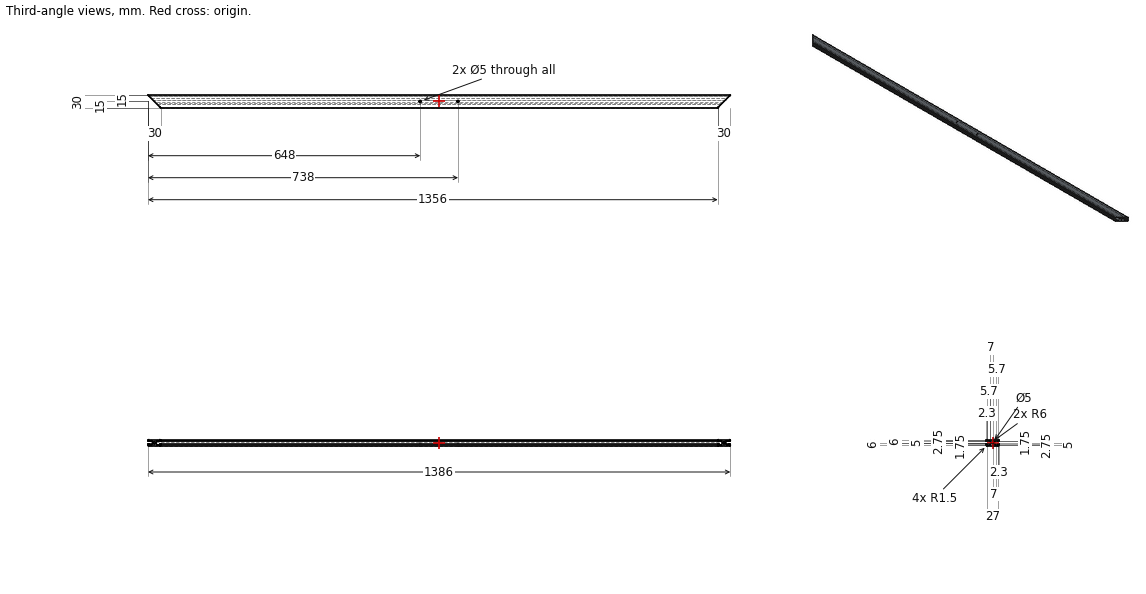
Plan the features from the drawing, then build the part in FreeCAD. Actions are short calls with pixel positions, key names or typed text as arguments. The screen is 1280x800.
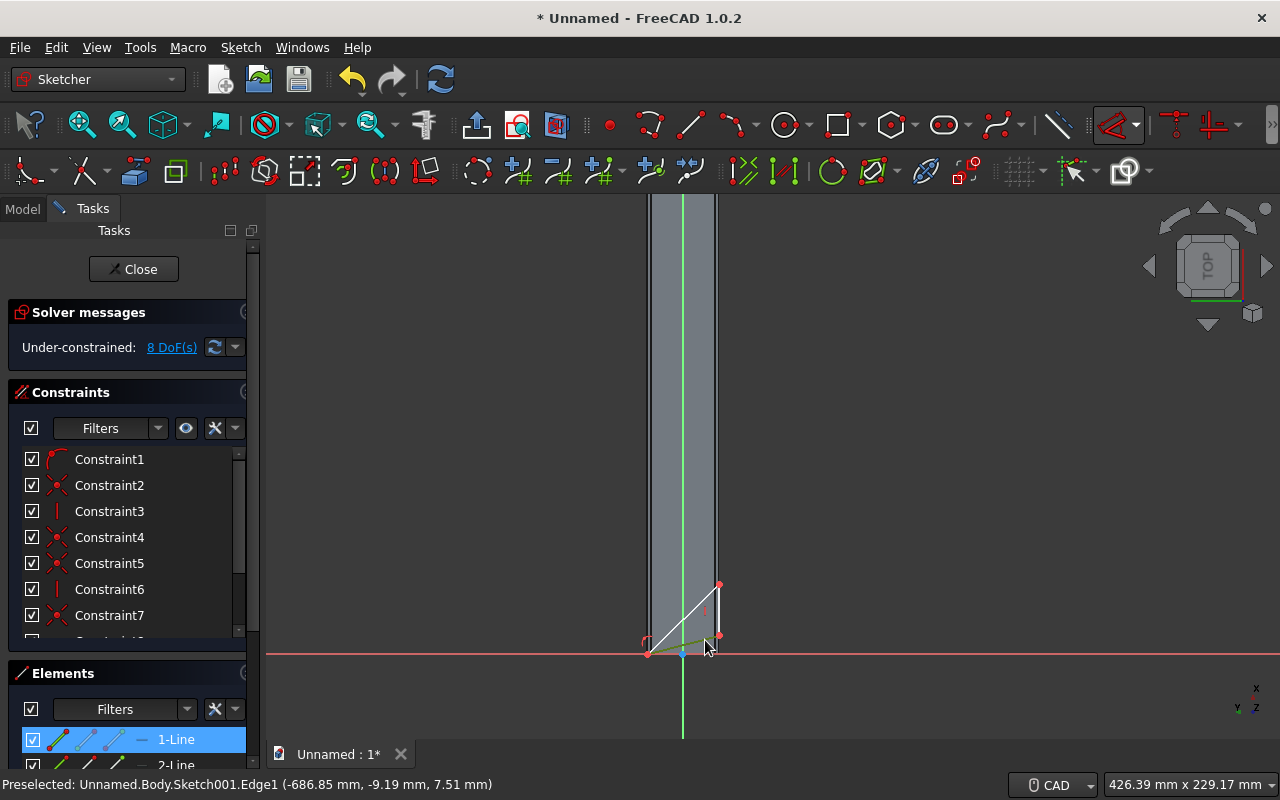
click(1240, 126)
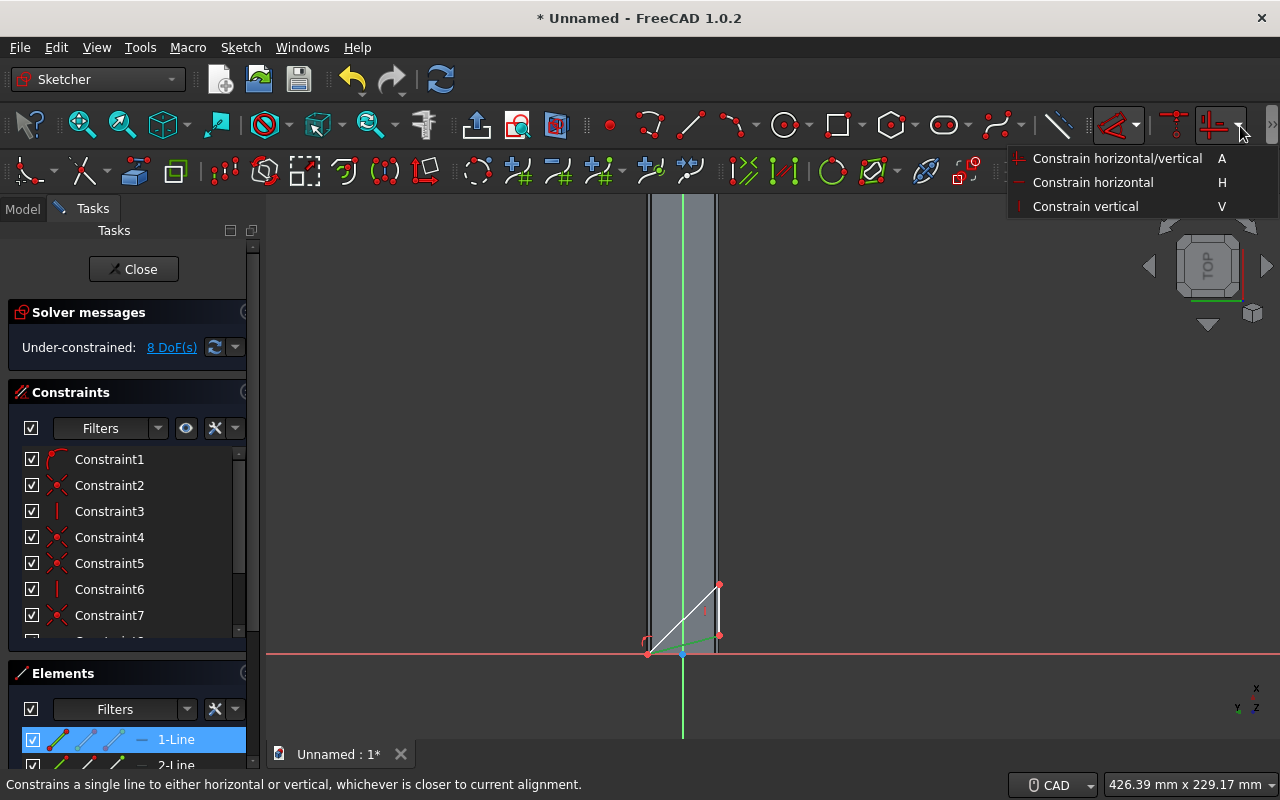
click(1143, 182)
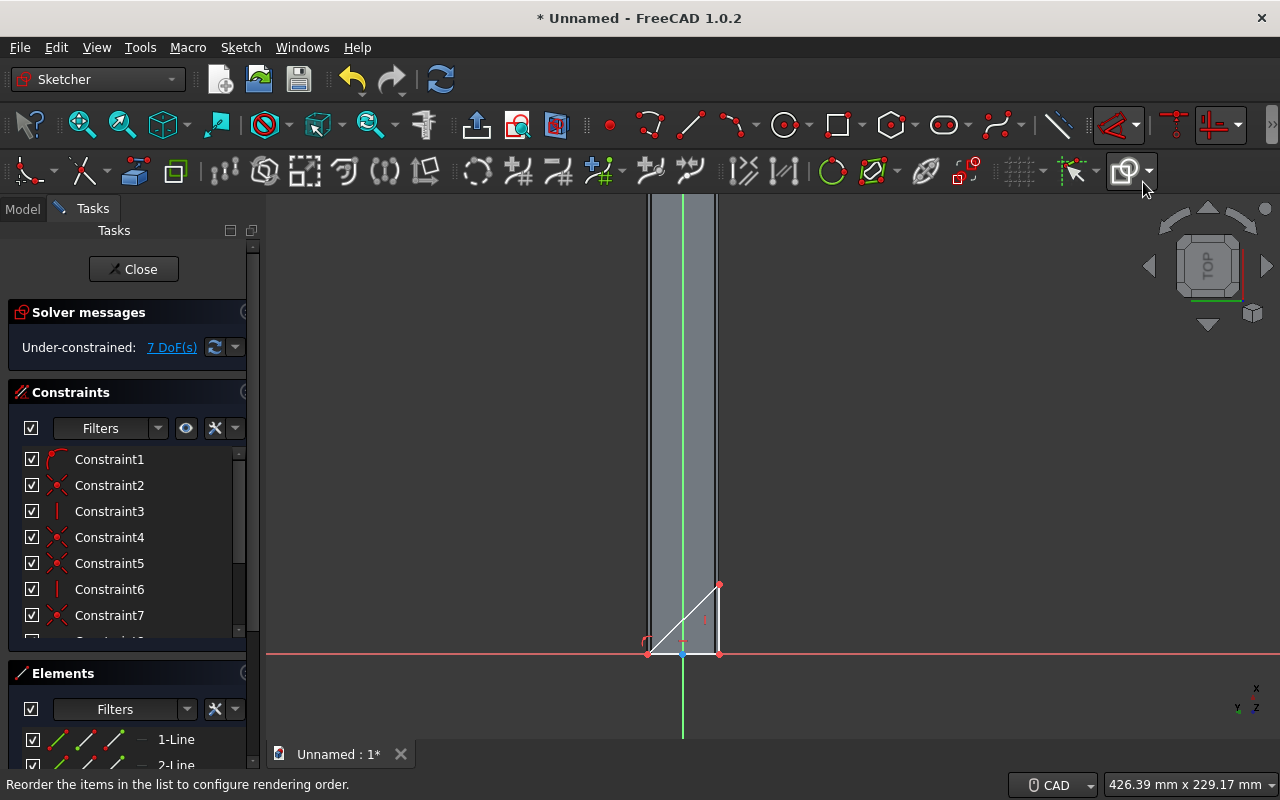
click(669, 654)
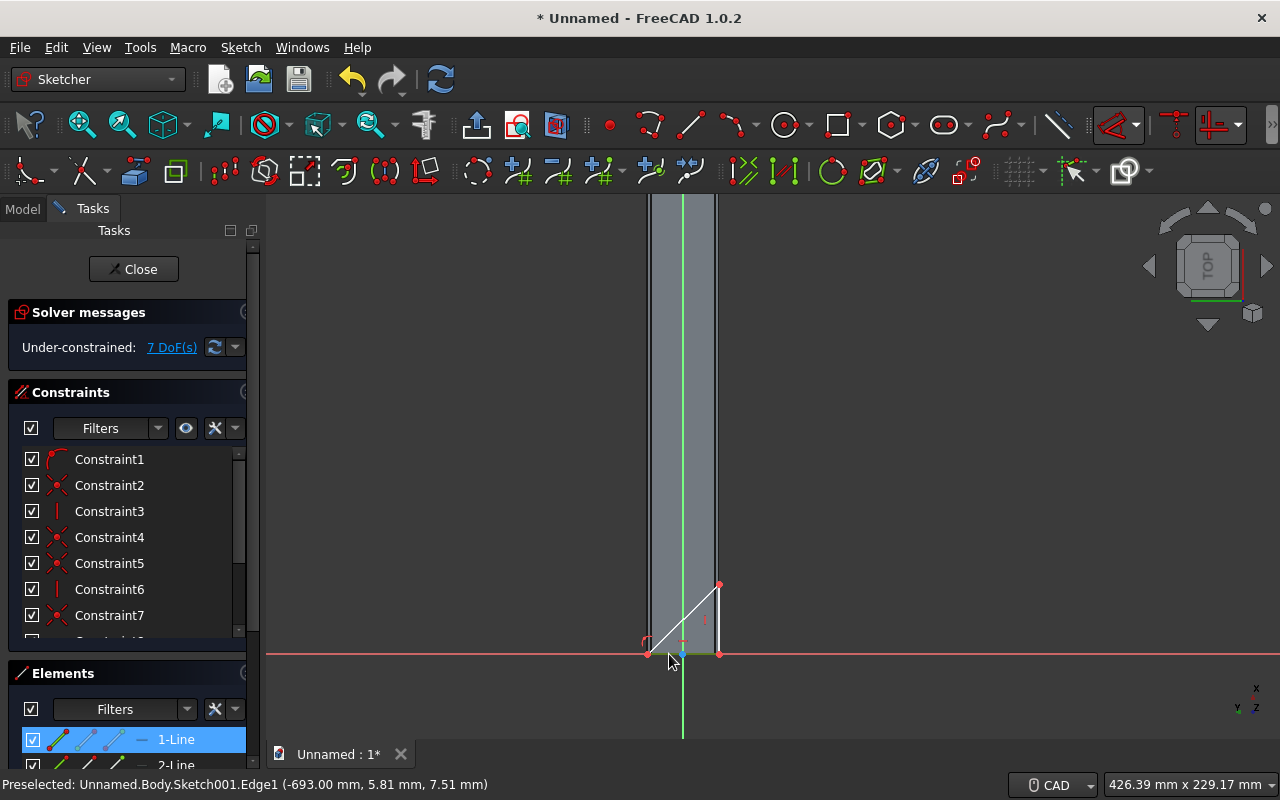
click(1138, 126)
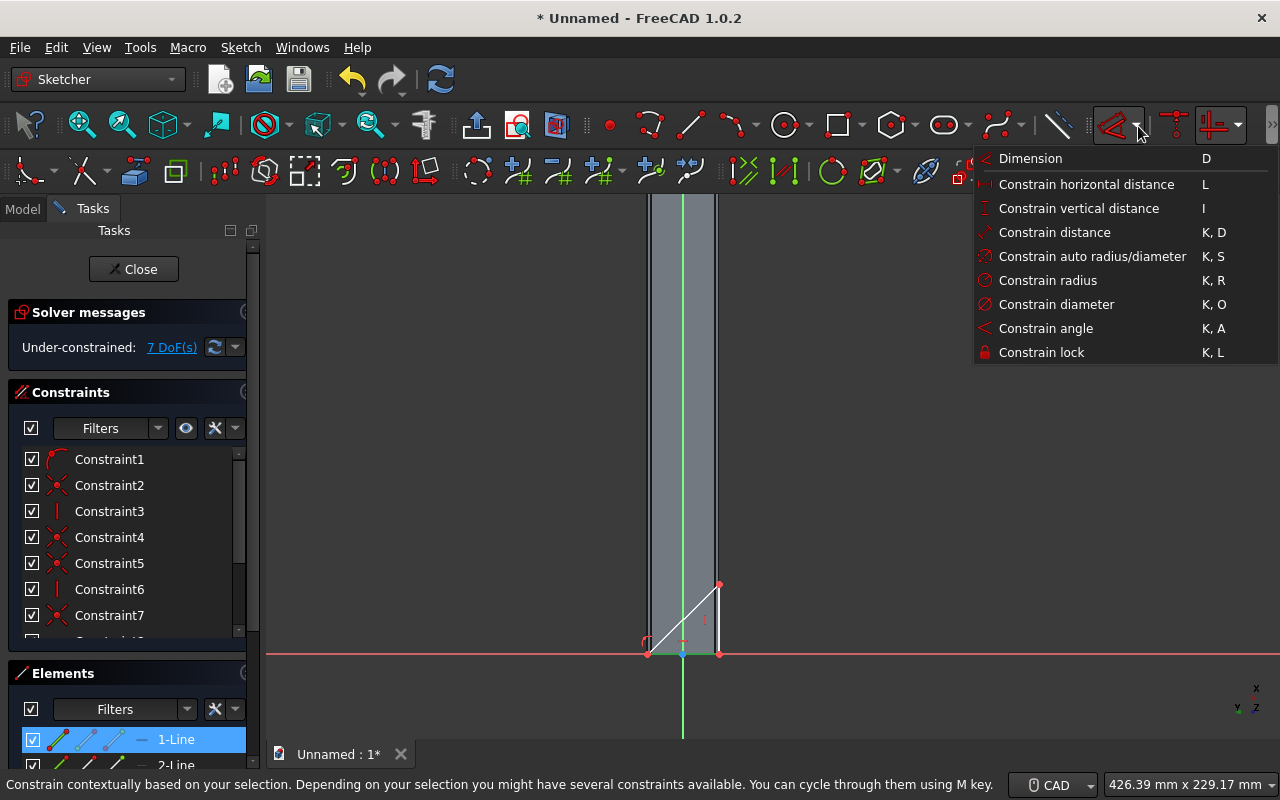
click(1126, 184)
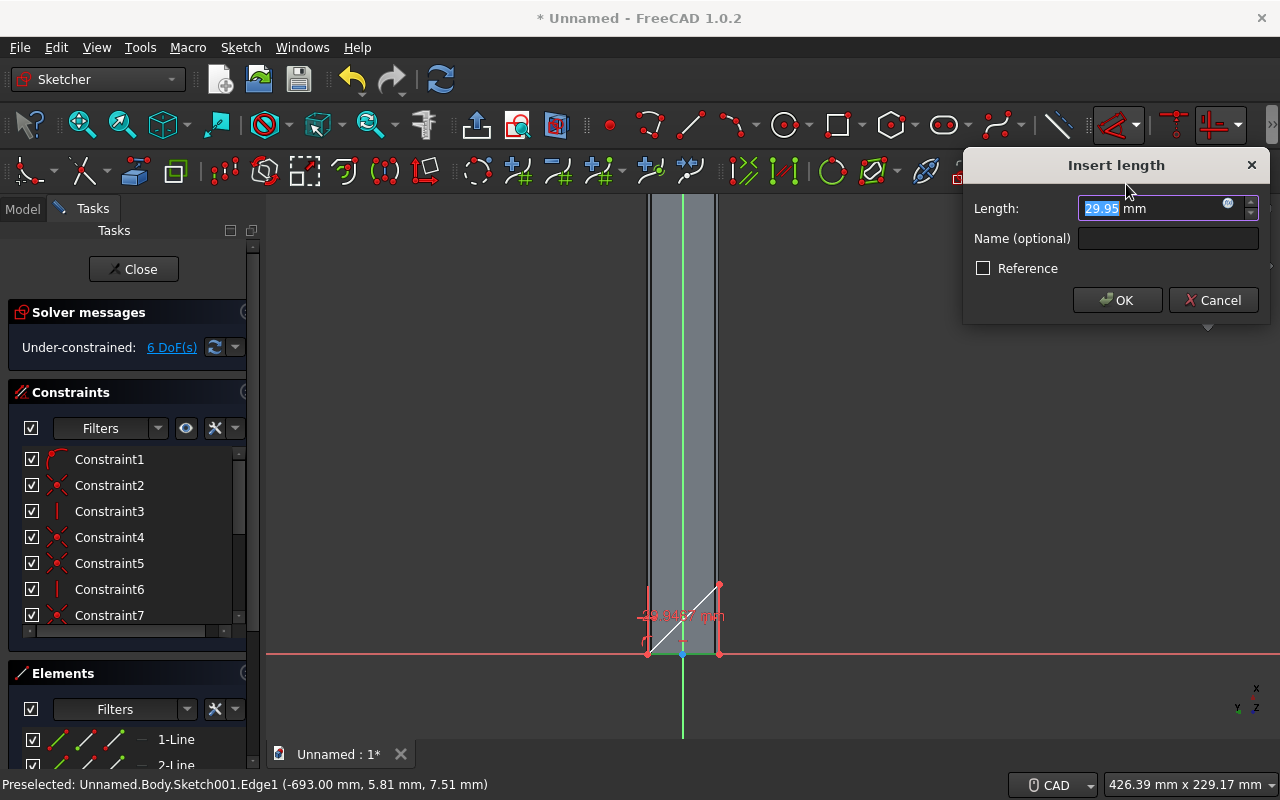
text(30)
key(Return)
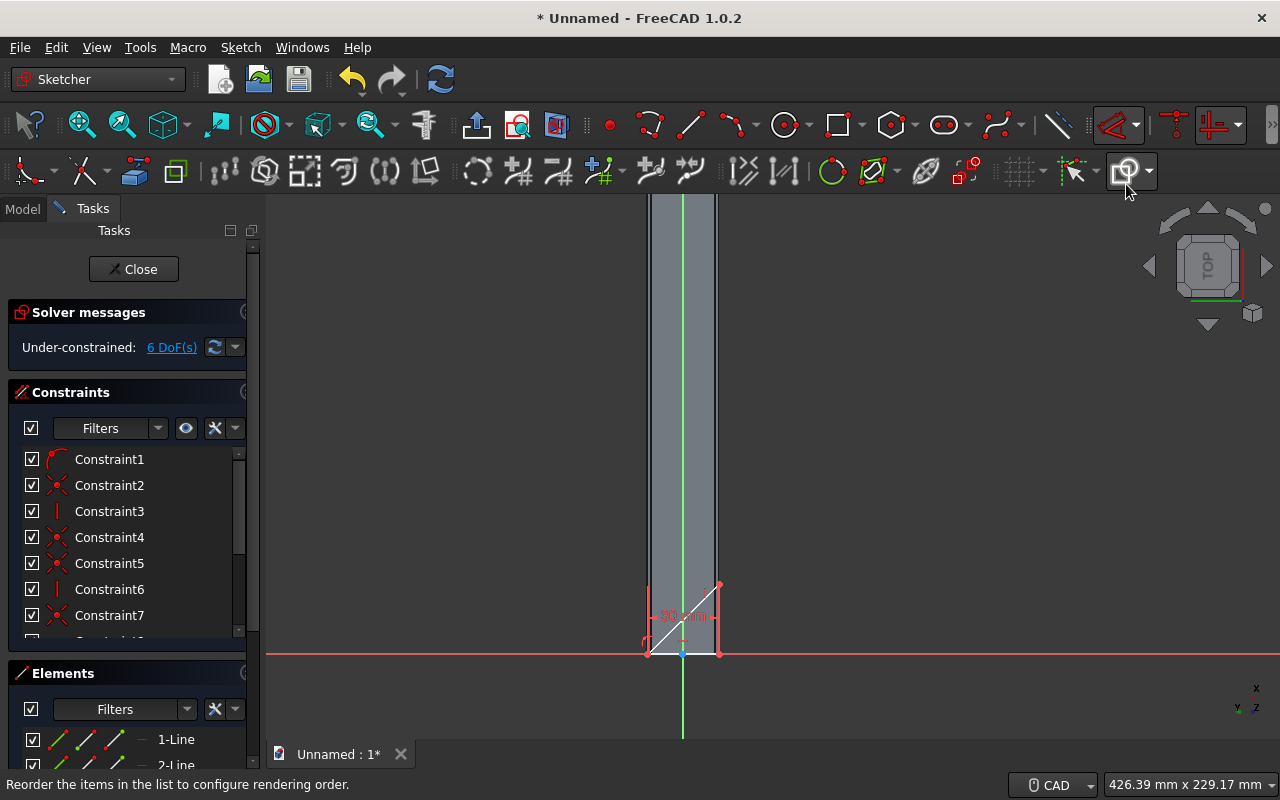
click(719, 633)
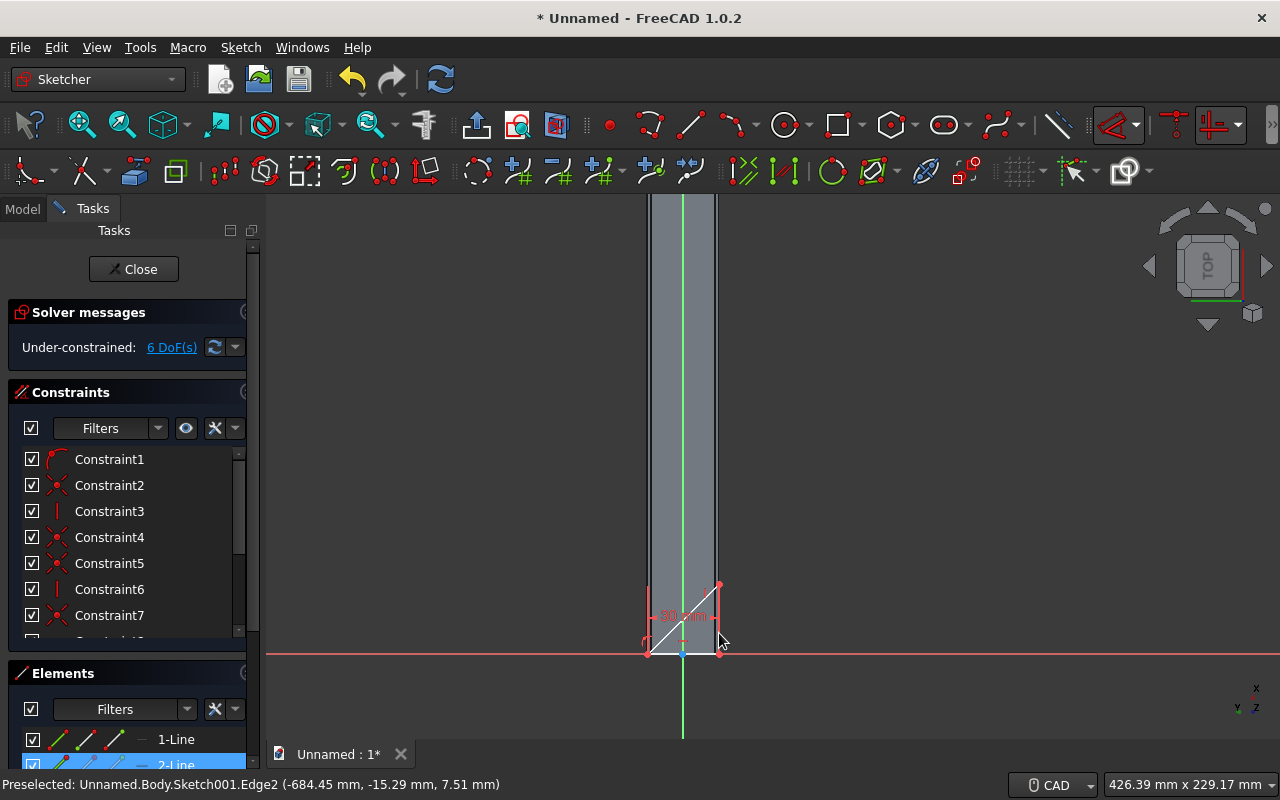
key(i)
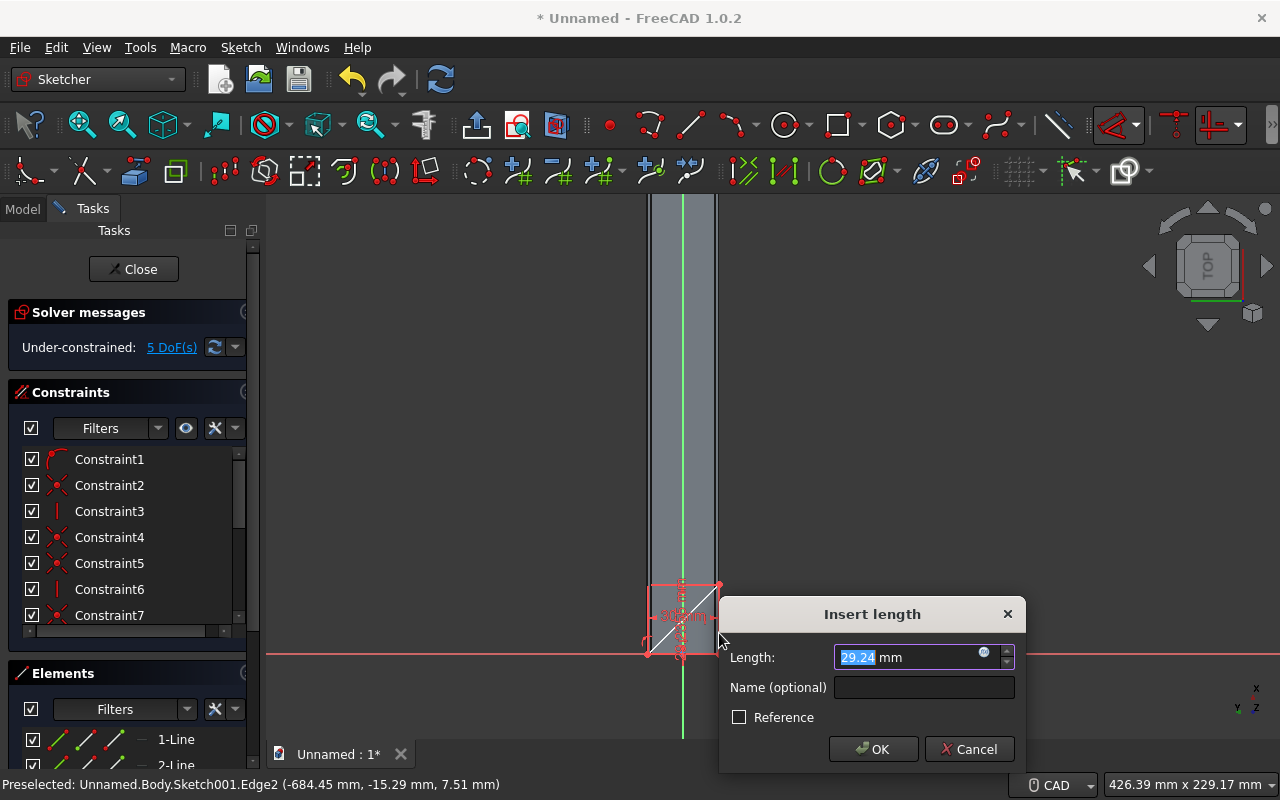
text(30)
key(Return)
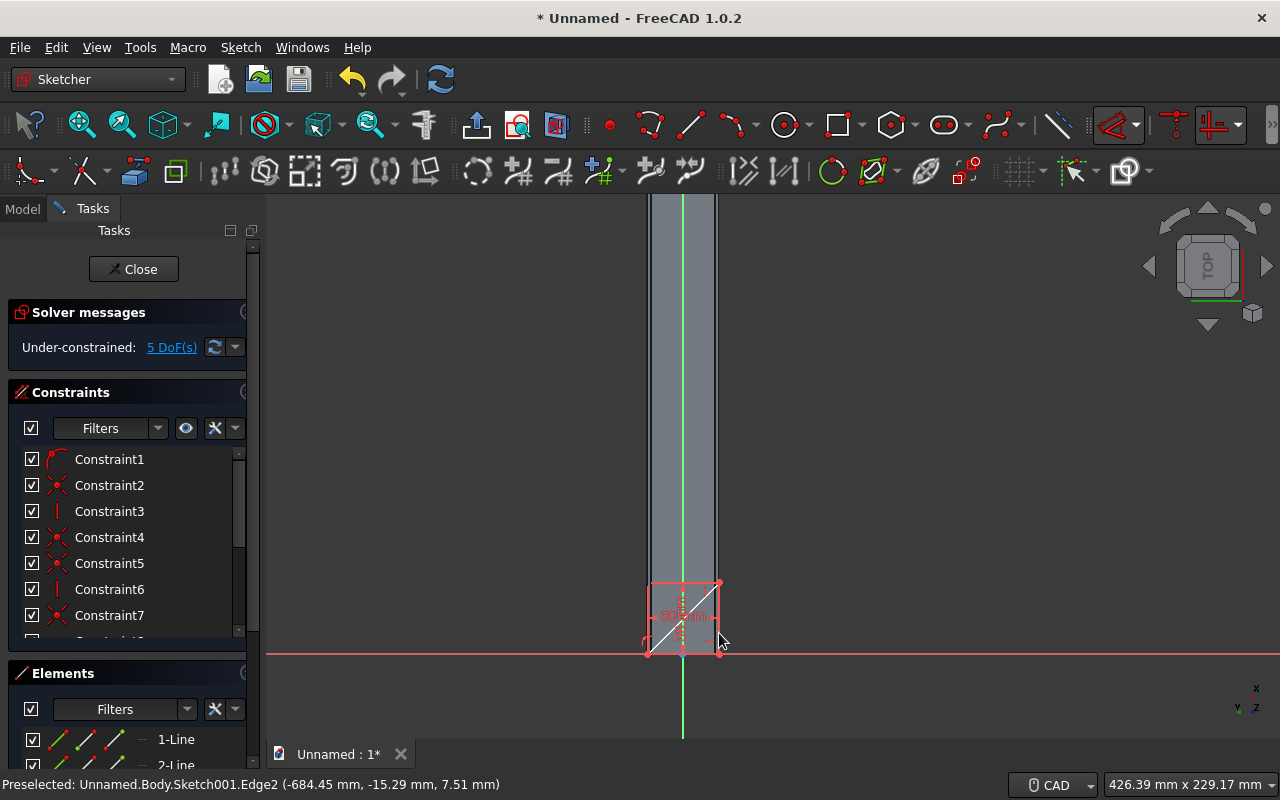
scroll(707, 648, down, 11)